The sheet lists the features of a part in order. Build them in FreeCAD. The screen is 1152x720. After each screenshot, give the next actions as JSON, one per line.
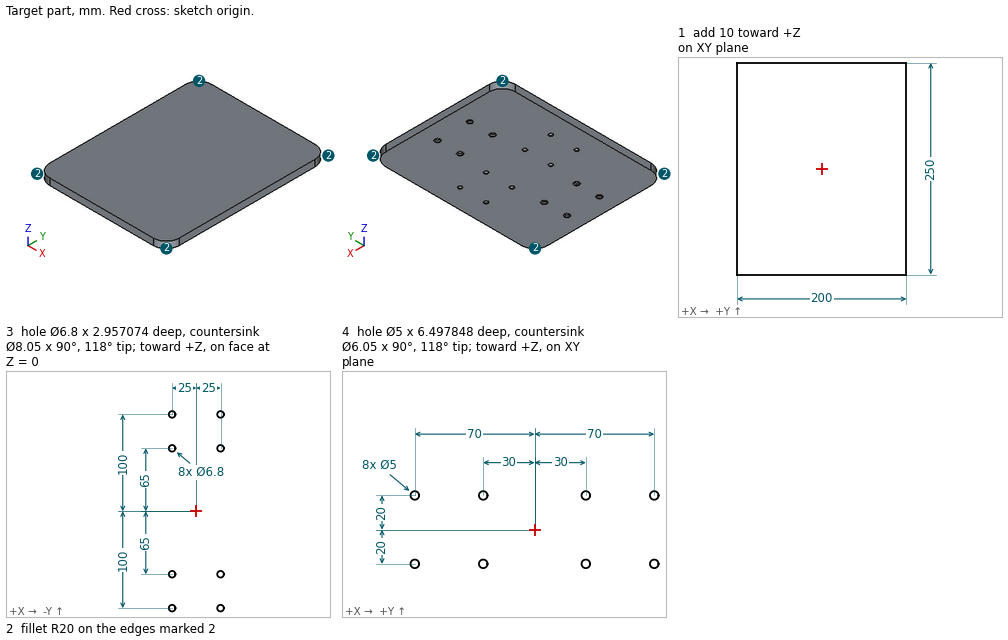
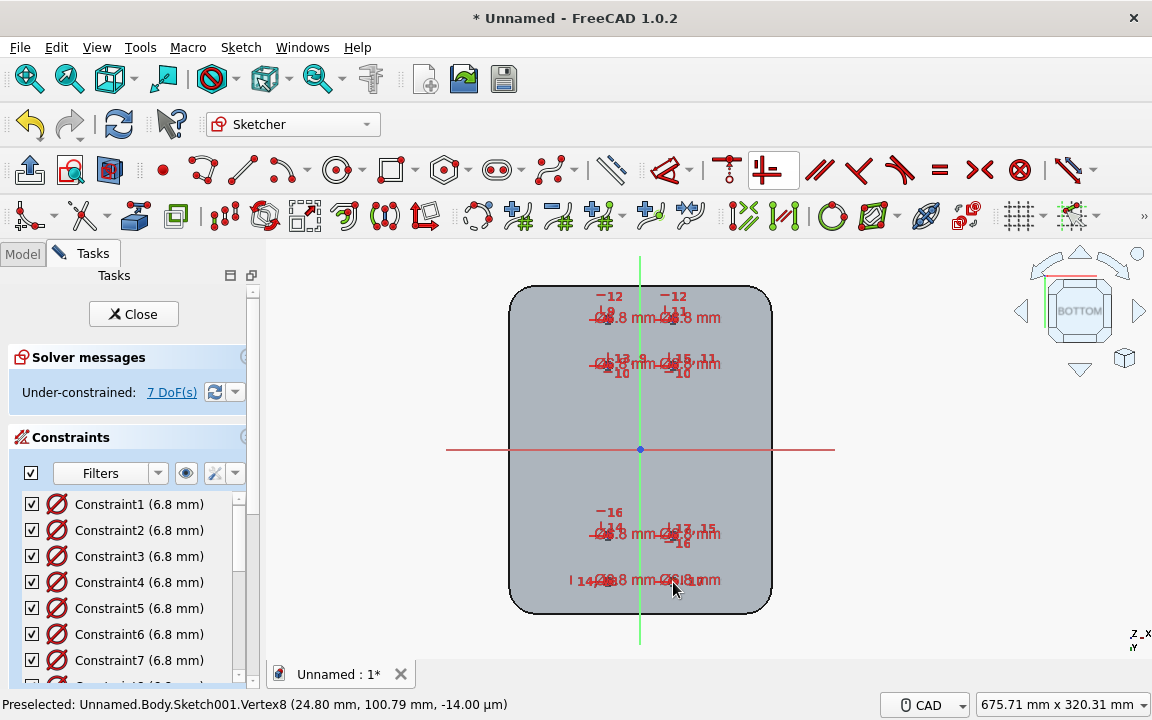
{"action": "left_click", "coordinate": [794, 170]}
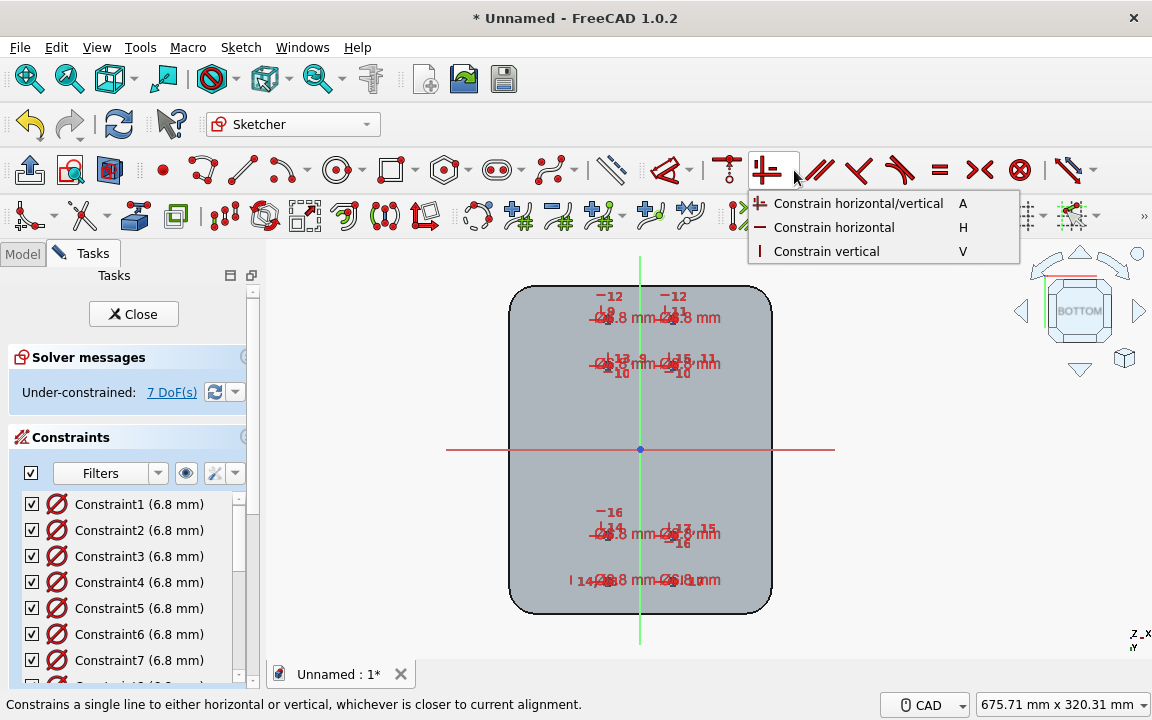
{"action": "left_click", "coordinate": [884, 227]}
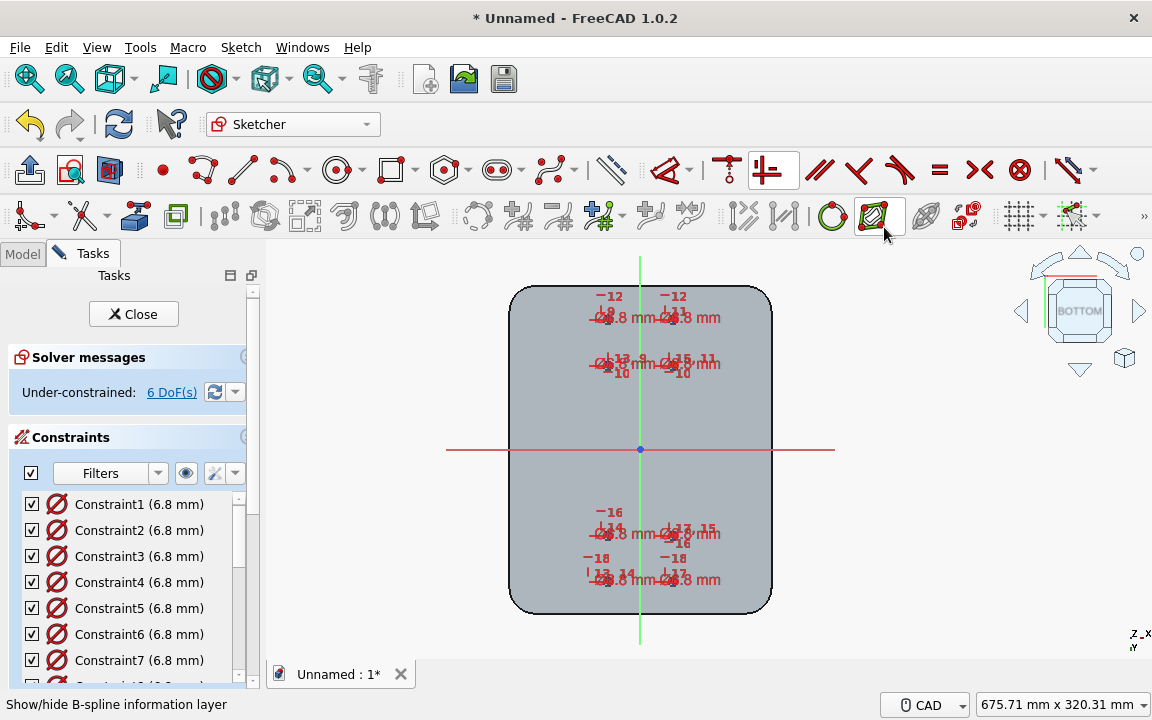
{"action": "left_click", "coordinate": [666, 170]}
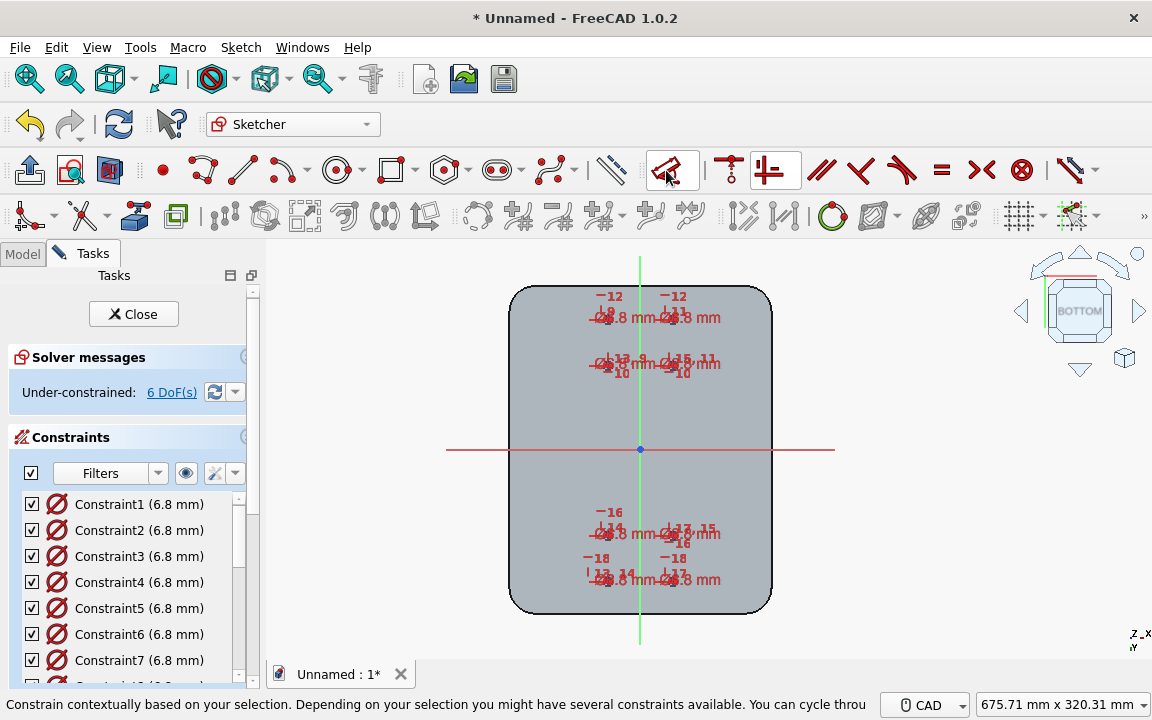
{"action": "left_click", "coordinate": [608, 320]}
{"action": "left_click", "coordinate": [624, 286]}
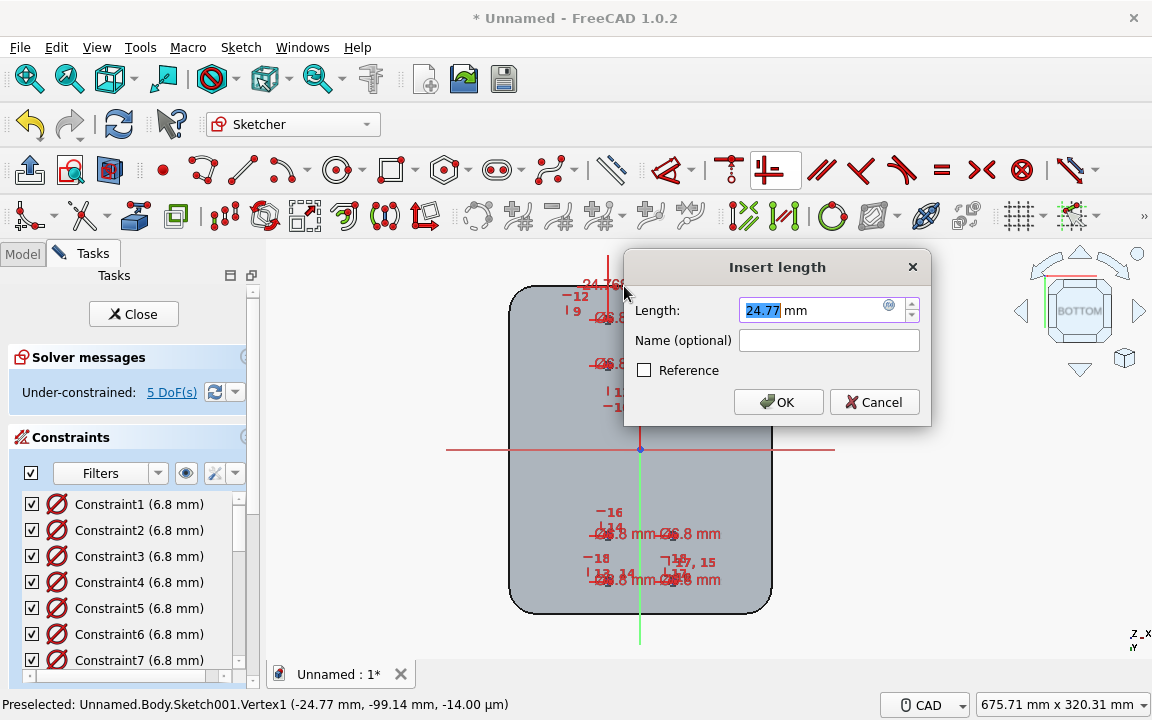
{"action": "type", "text": "25"}
{"action": "key", "text": "Return"}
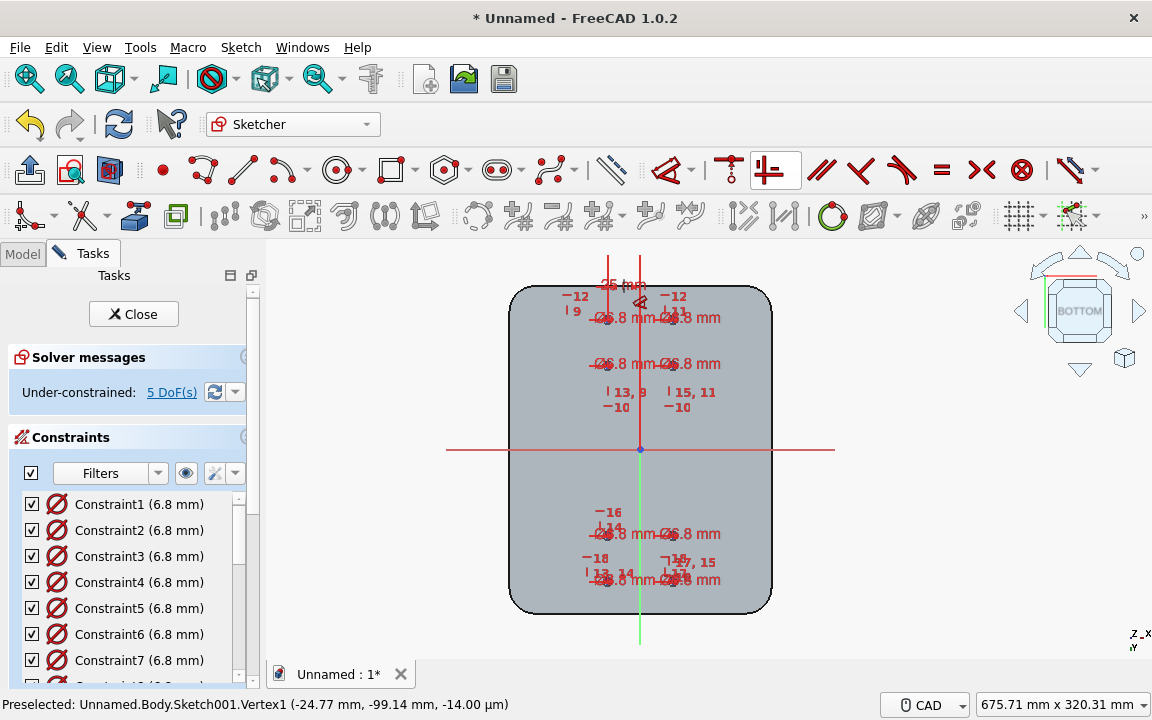
{"action": "left_click", "coordinate": [608, 366]}
{"action": "left_click", "coordinate": [574, 408]}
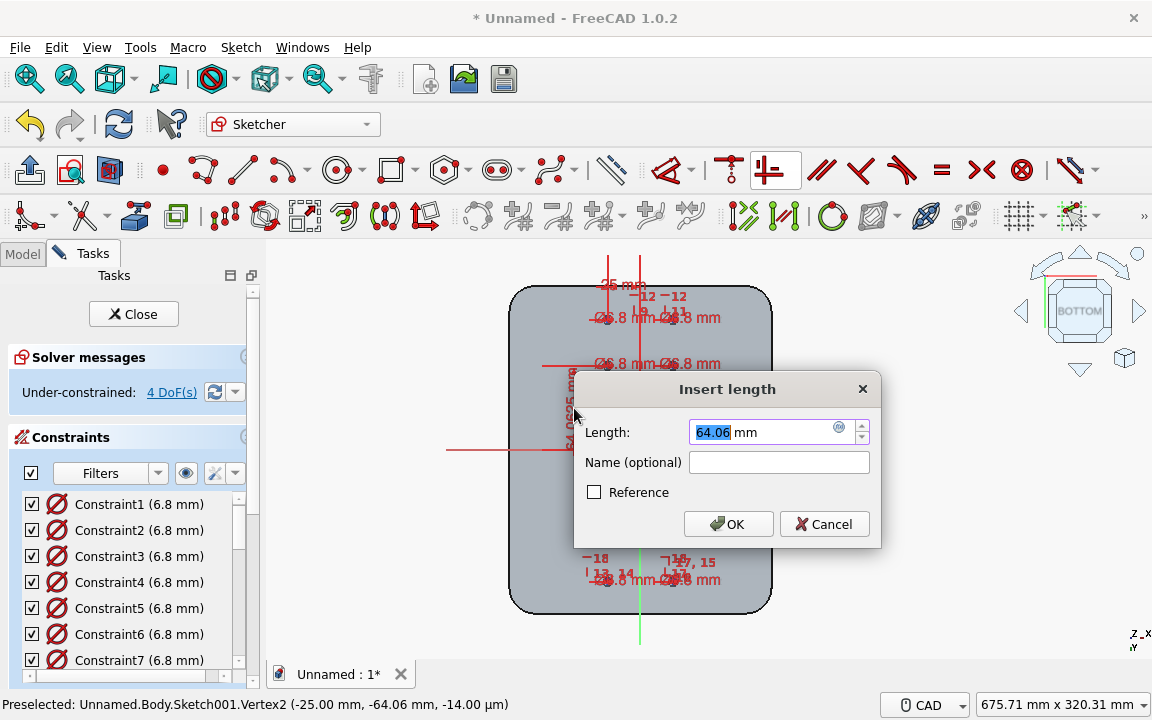
{"action": "type", "text": "65"}
{"action": "key", "text": "Return"}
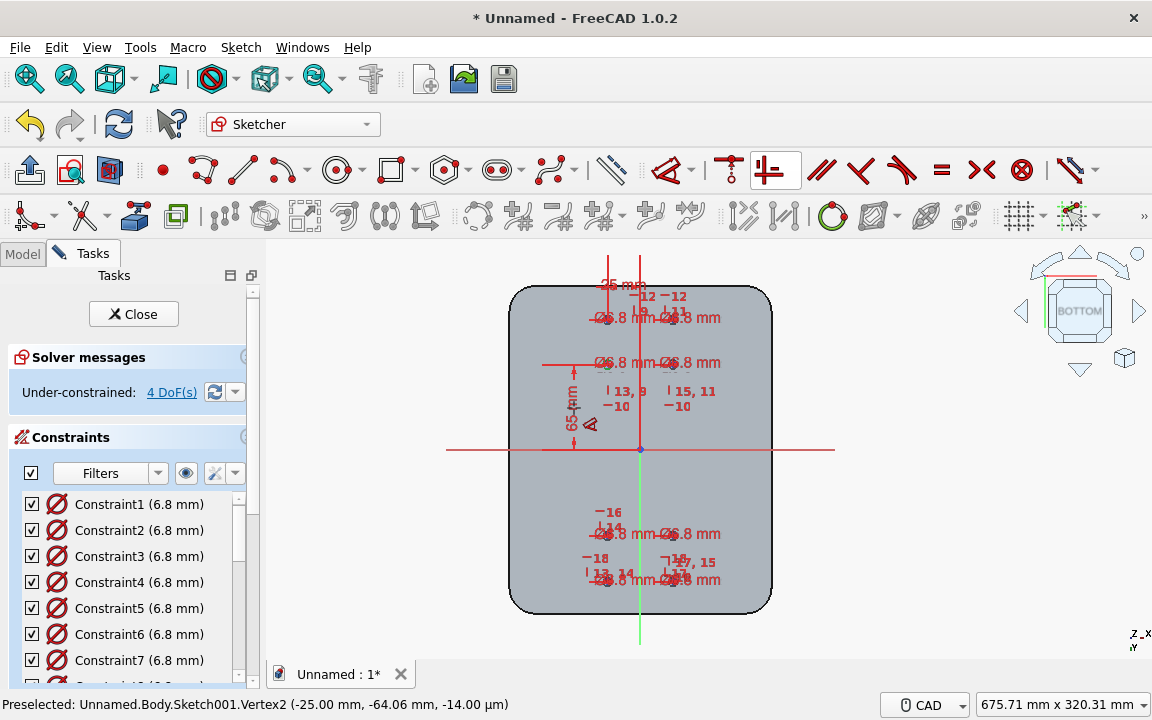
{"action": "left_click", "coordinate": [673, 365]}
{"action": "left_click", "coordinate": [657, 331]}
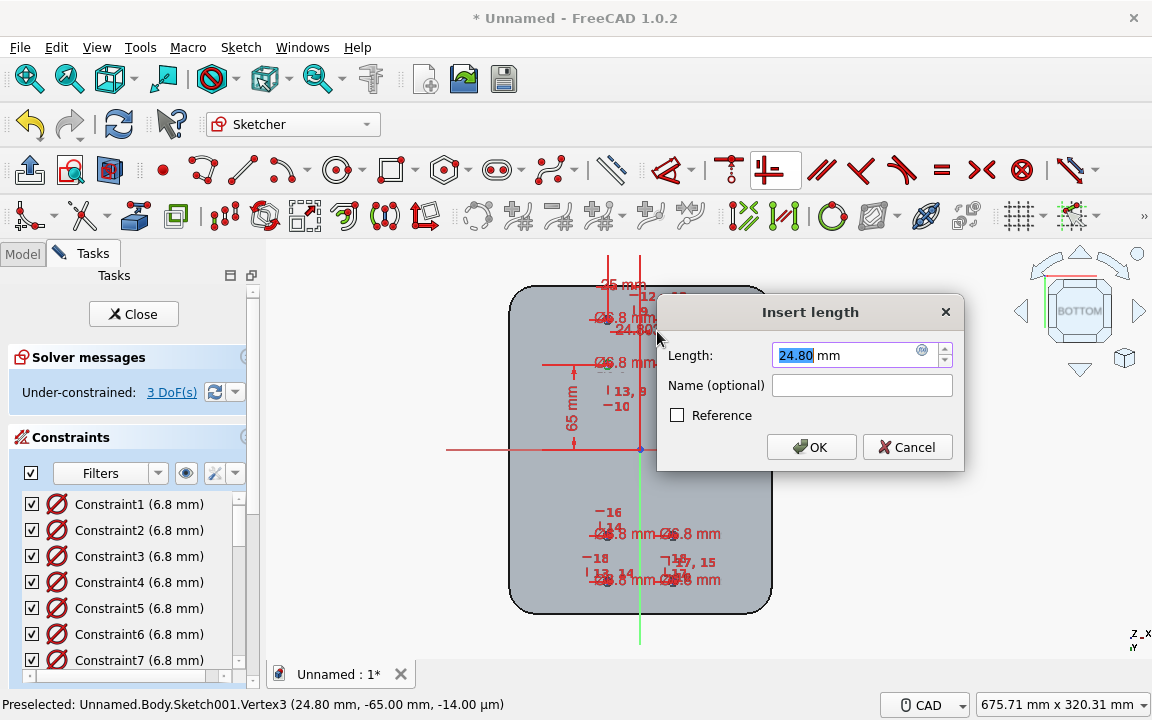
{"action": "type", "text": "25"}
{"action": "key", "text": "Return"}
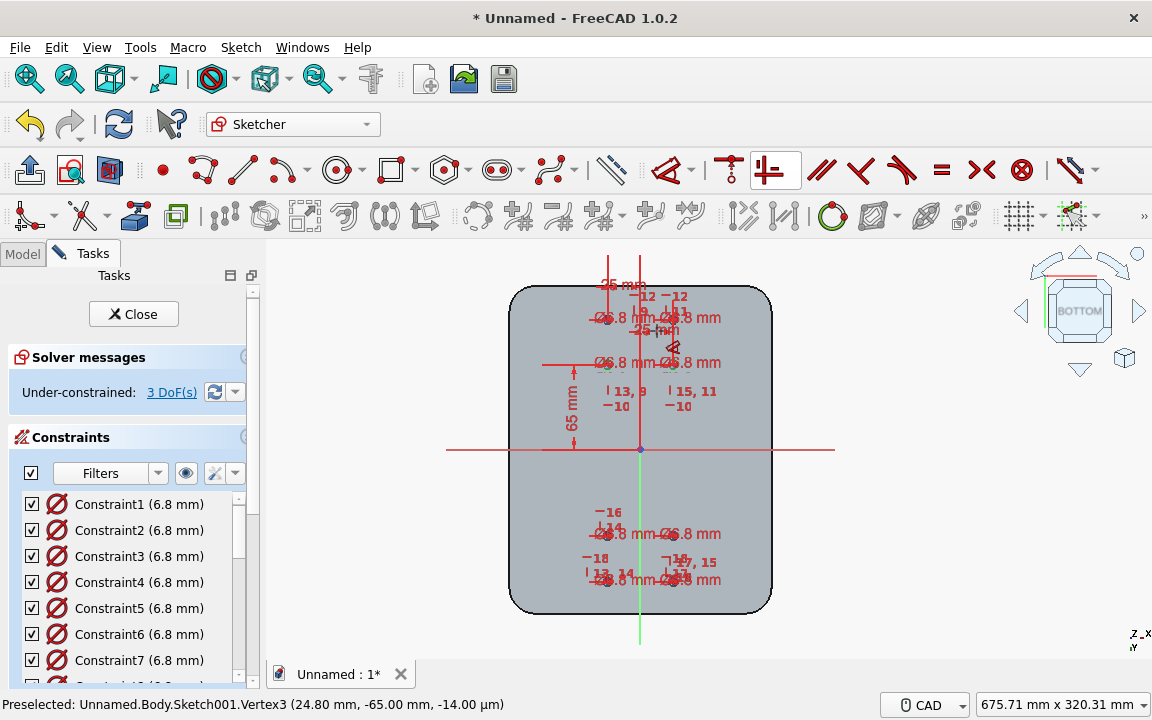
{"action": "left_click", "coordinate": [608, 536]}
{"action": "left_click", "coordinate": [574, 493]}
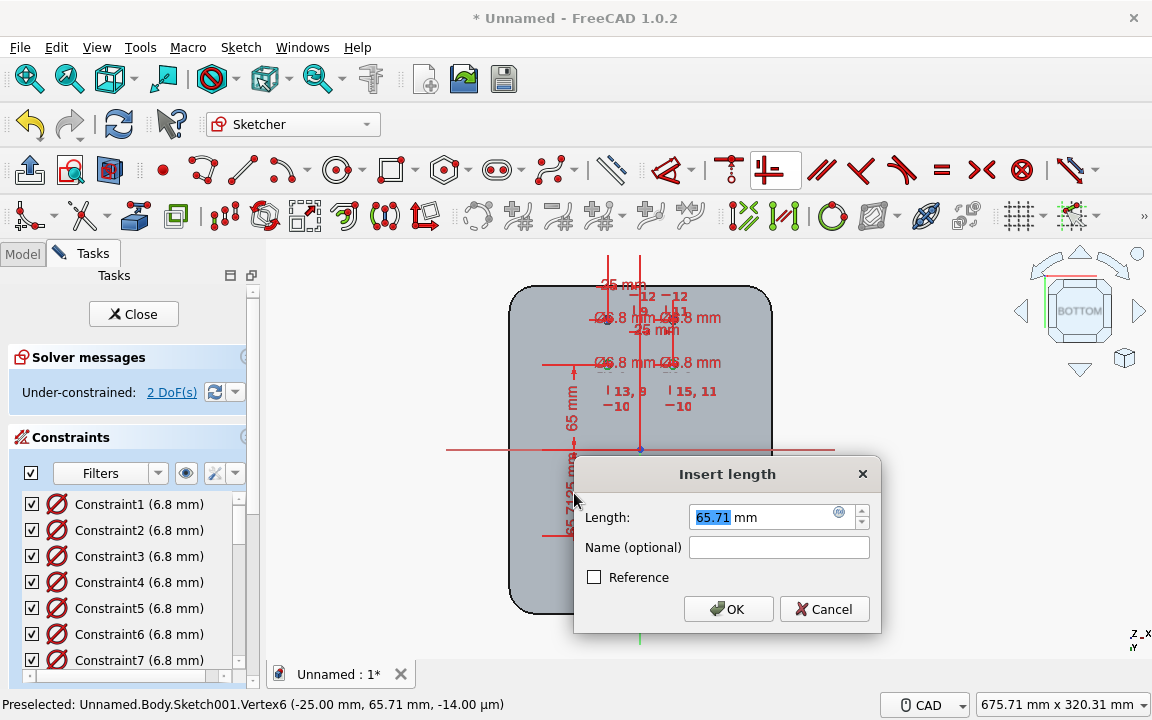
{"action": "type", "text": "65"}
{"action": "key", "text": "Return"}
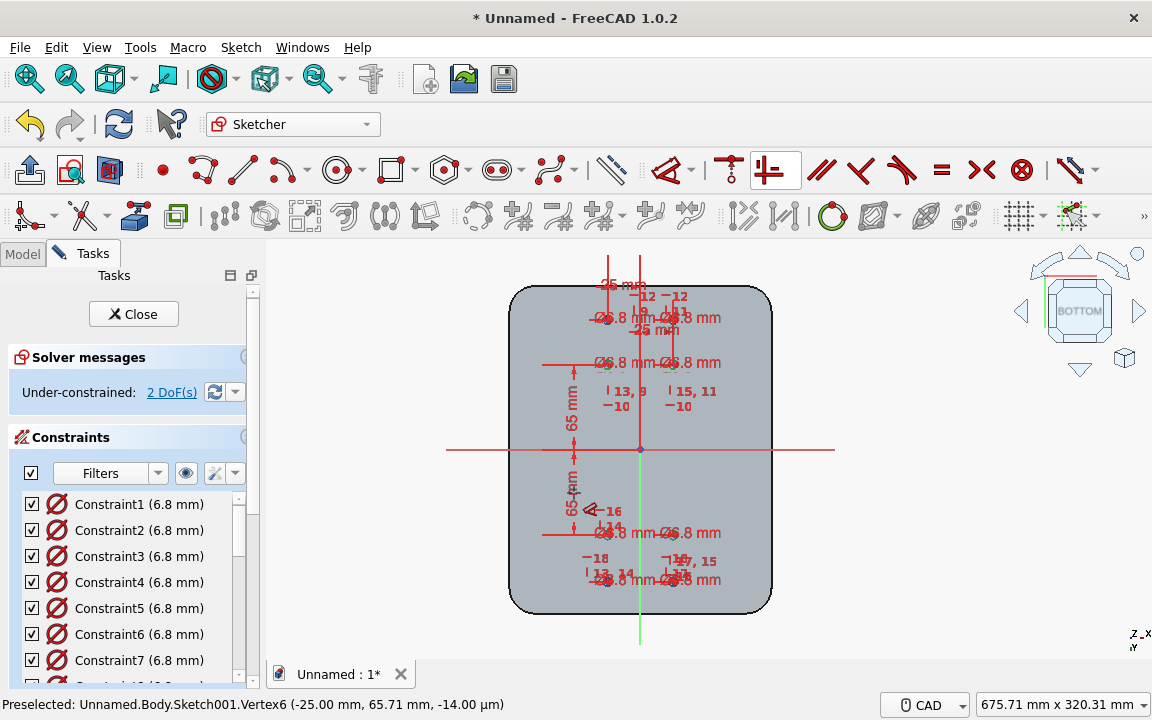
{"action": "left_click", "coordinate": [608, 320]}
{"action": "left_click", "coordinate": [574, 385]}